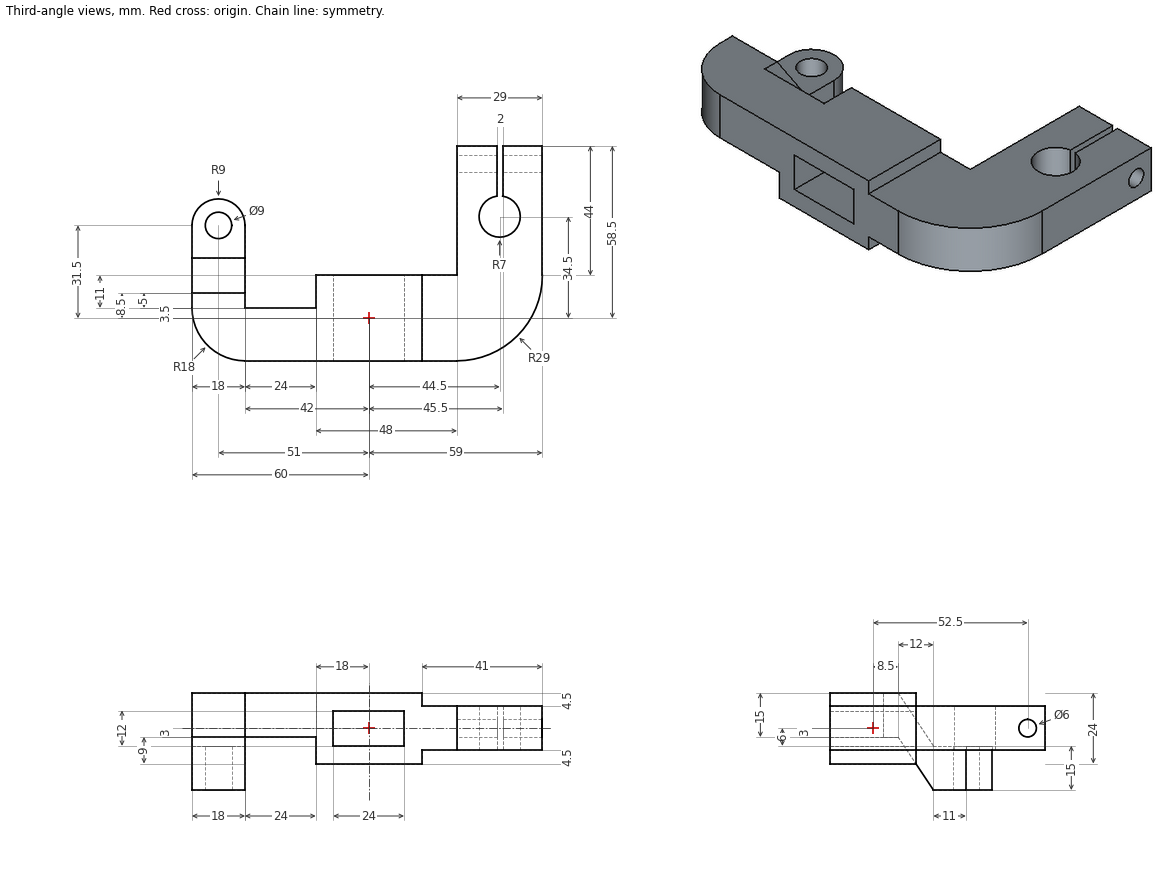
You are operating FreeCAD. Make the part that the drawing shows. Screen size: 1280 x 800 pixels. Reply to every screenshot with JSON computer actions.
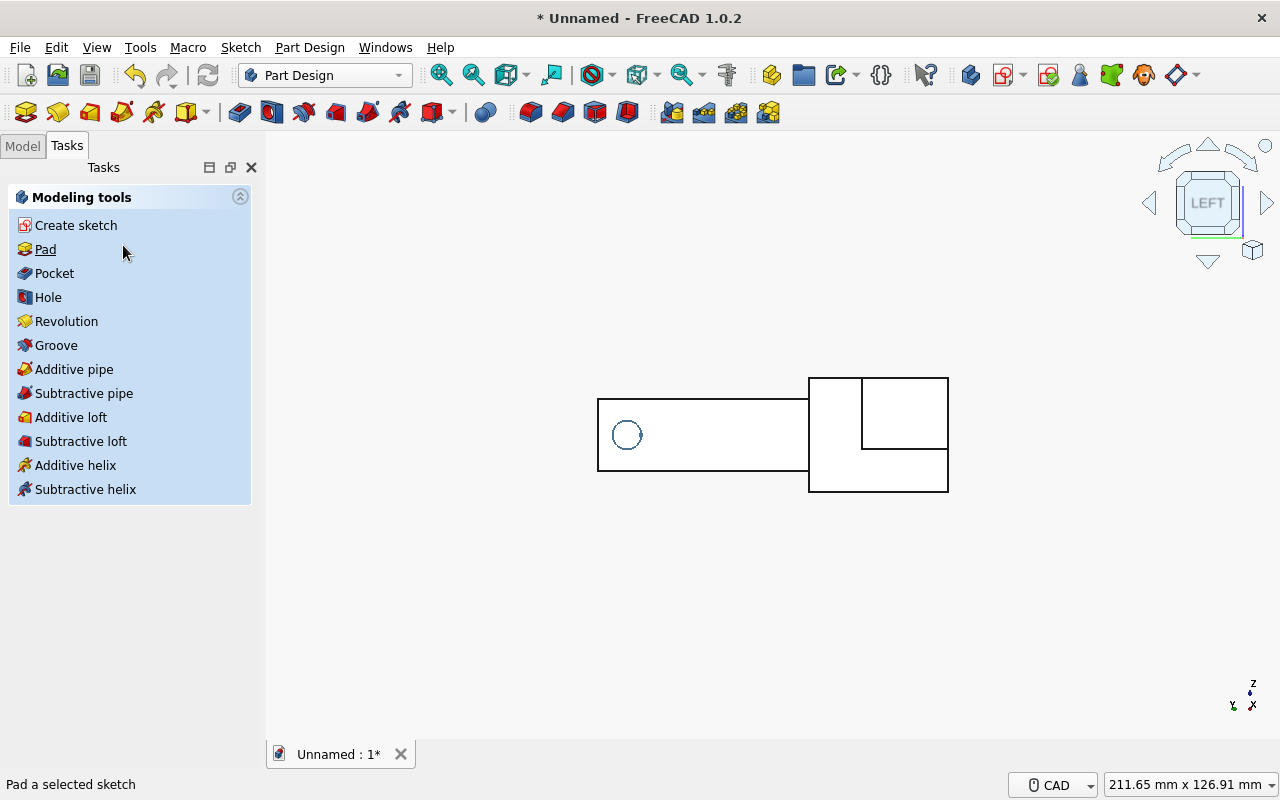
{"action": "left_click", "coordinate": [240, 112]}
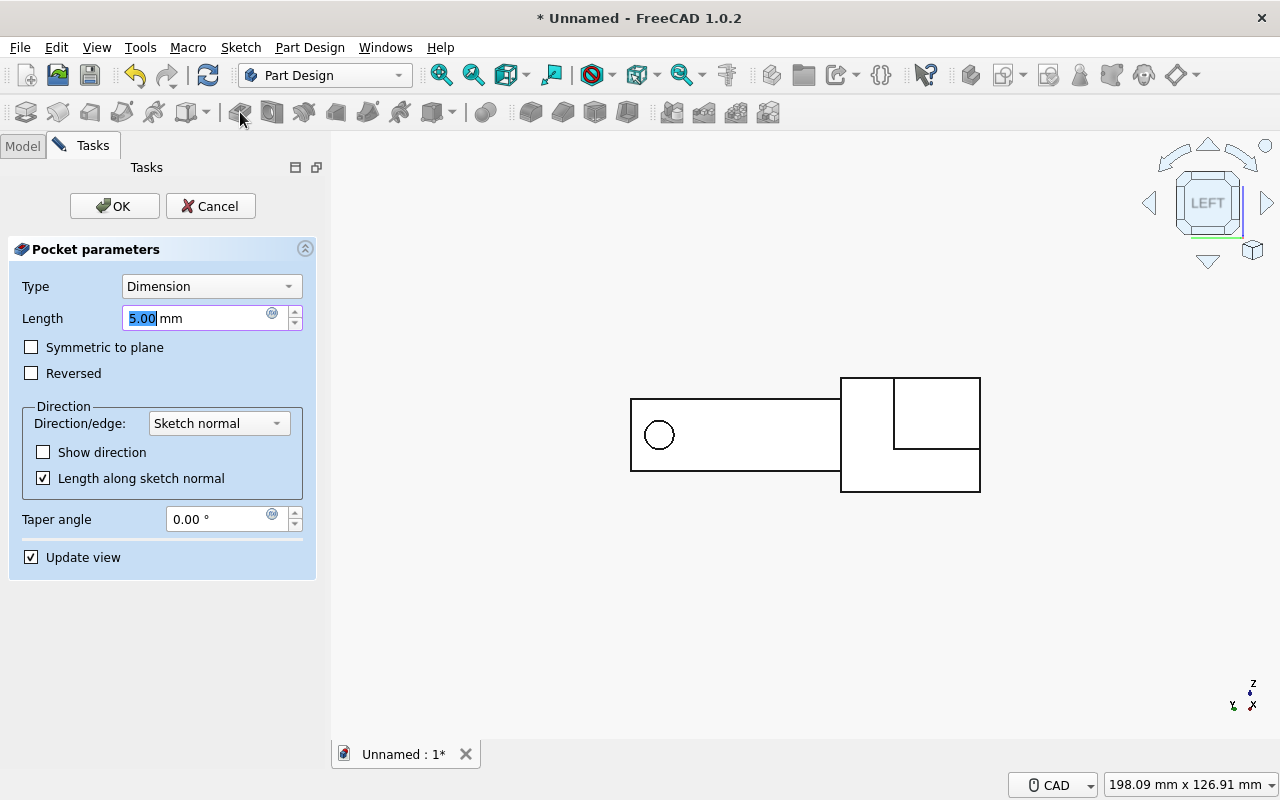
{"action": "left_click", "coordinate": [212, 286]}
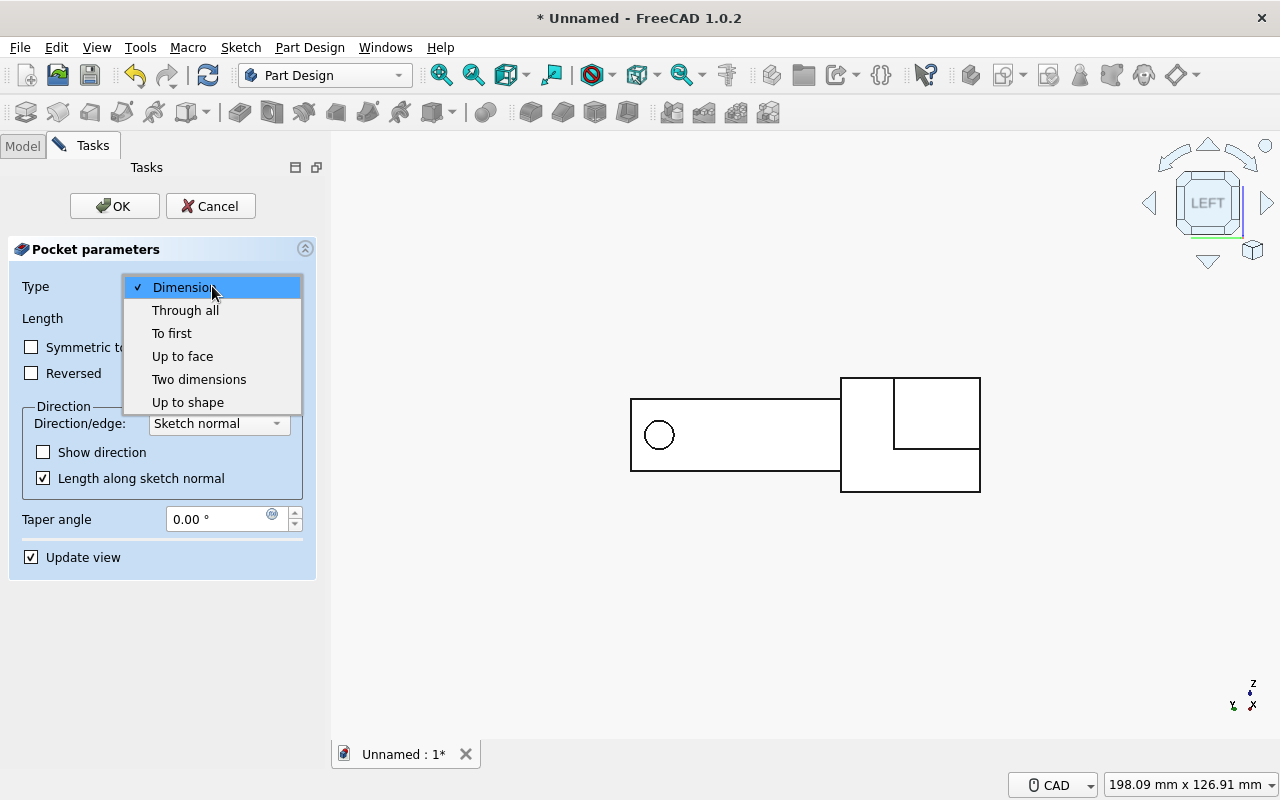
{"action": "left_click", "coordinate": [212, 310]}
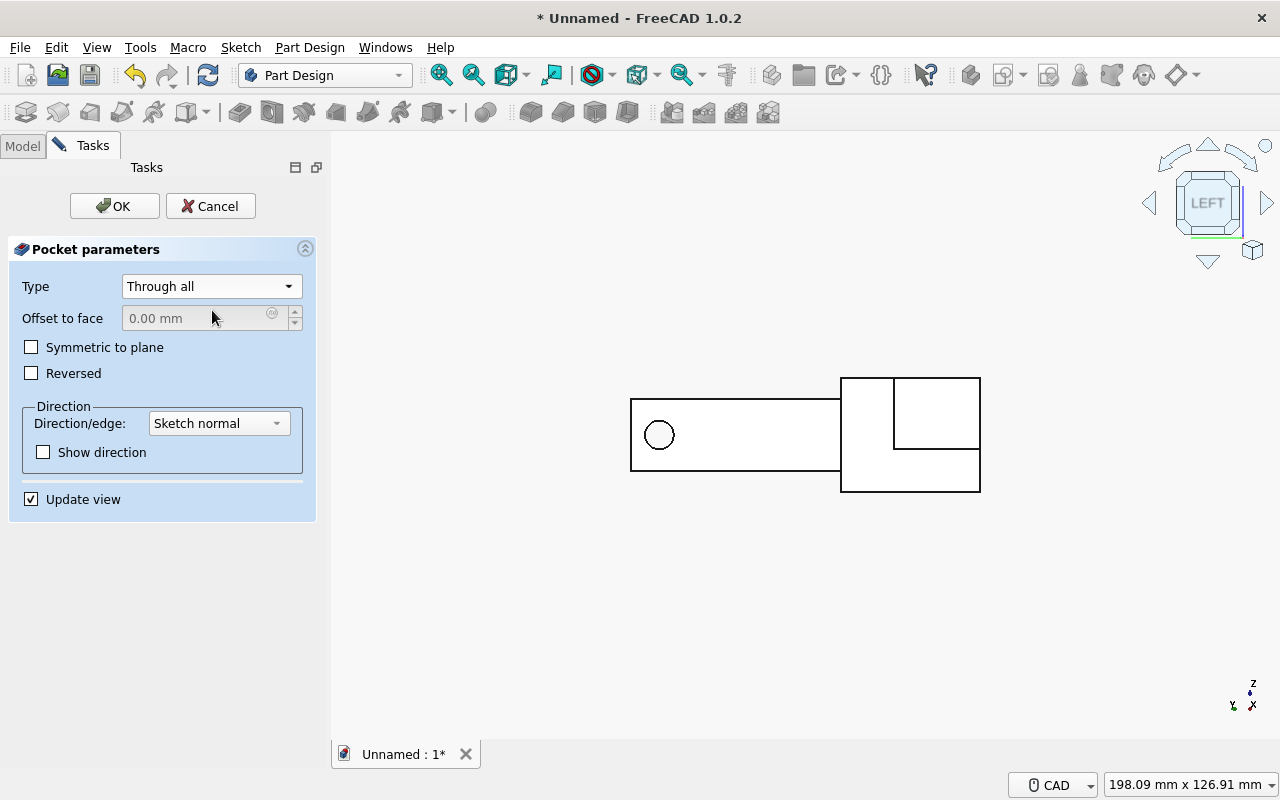
{"action": "left_click", "coordinate": [115, 206]}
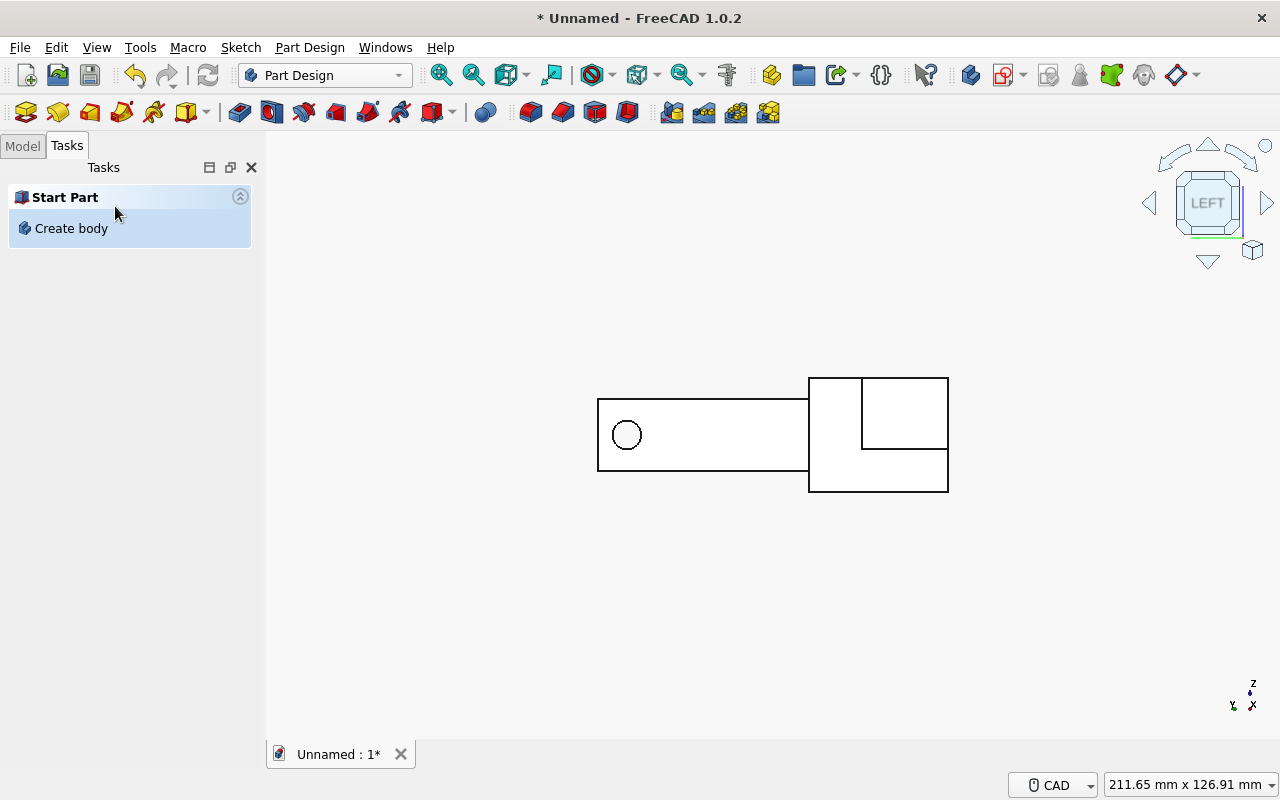
{"action": "left_click", "coordinate": [442, 76]}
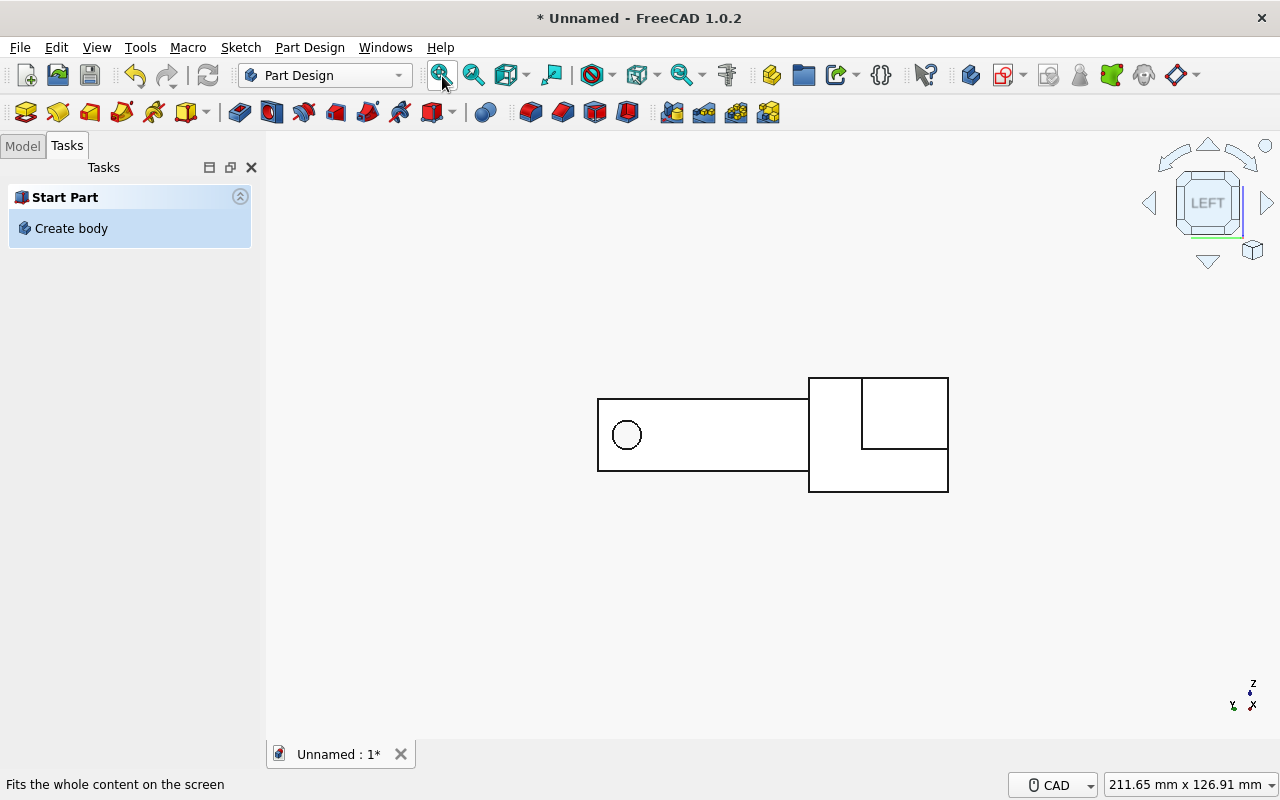
{"action": "key", "text": "0"}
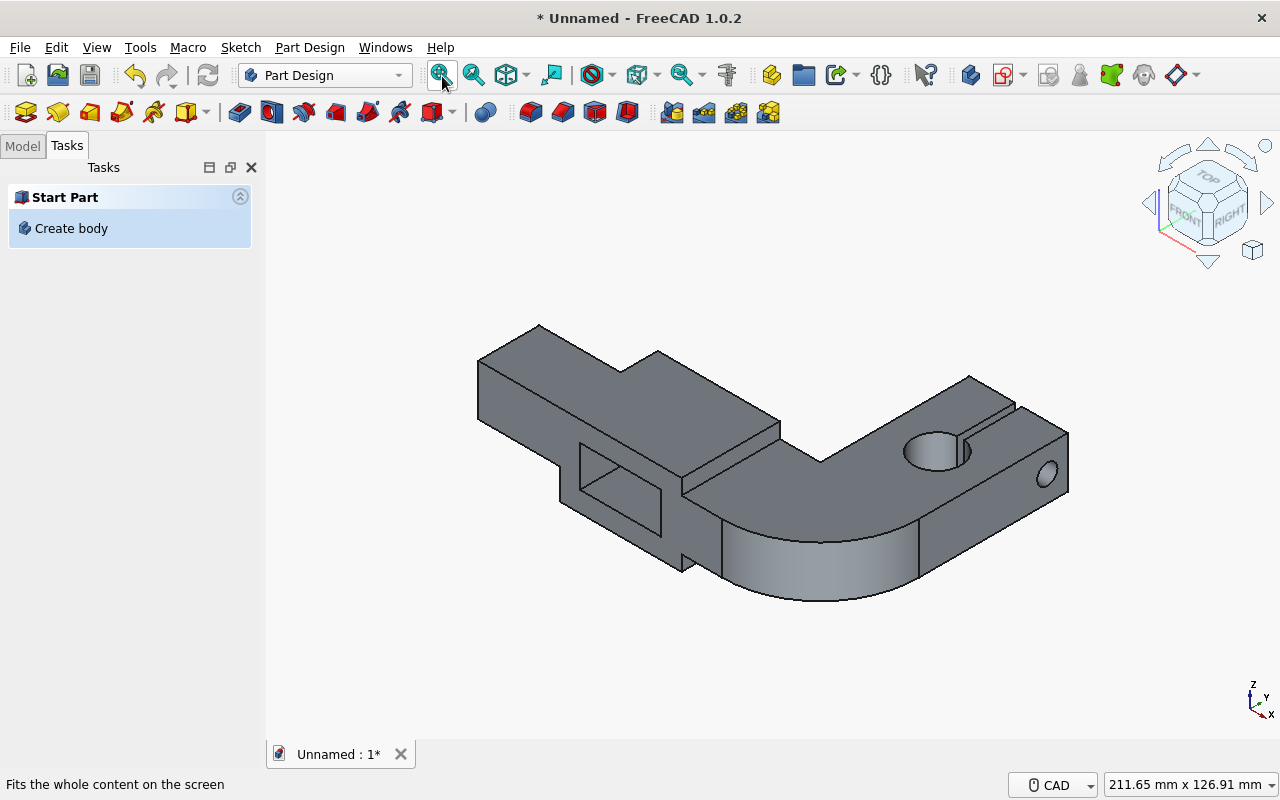
{"action": "left_click", "coordinate": [658, 407]}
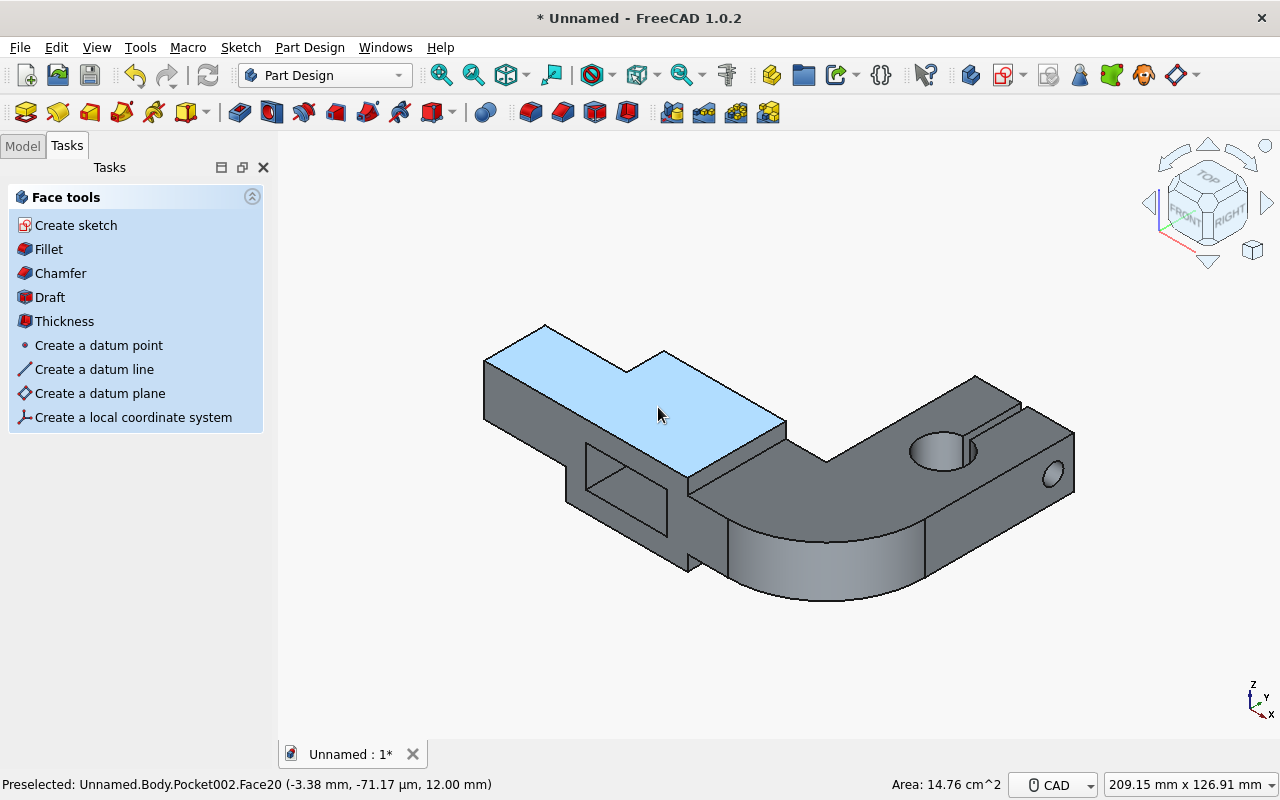
{"action": "left_click", "coordinate": [1004, 76]}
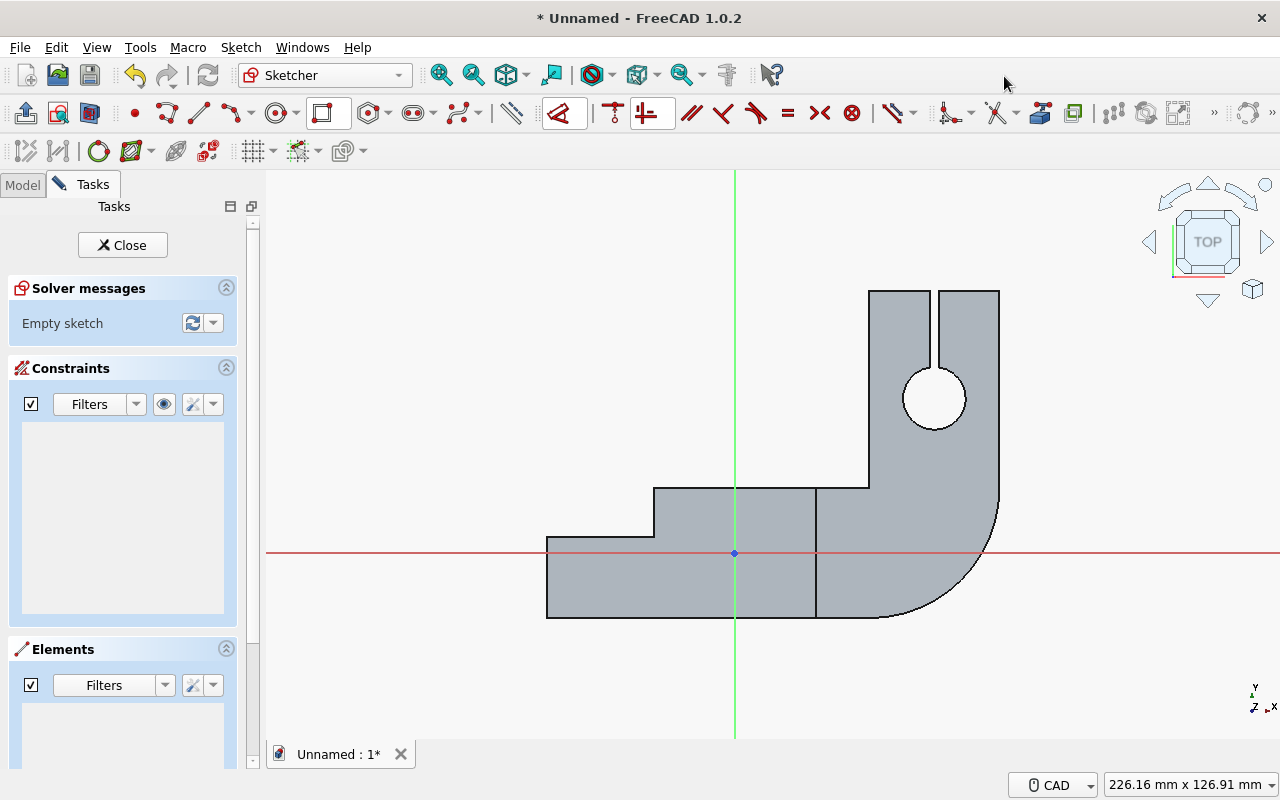
{"action": "scroll", "coordinate": [421, 615], "scroll_direction": "up", "scroll_amount": 6}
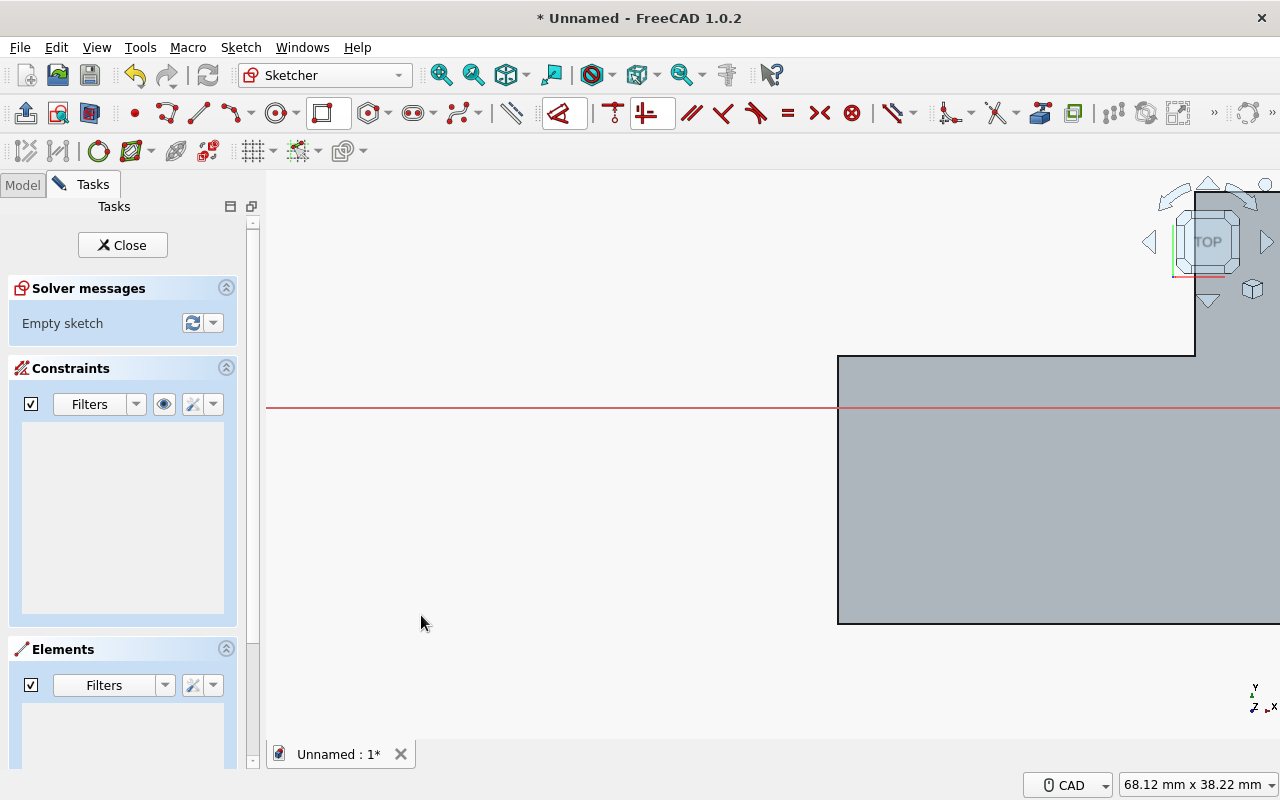
{"action": "left_click", "coordinate": [168, 114]}